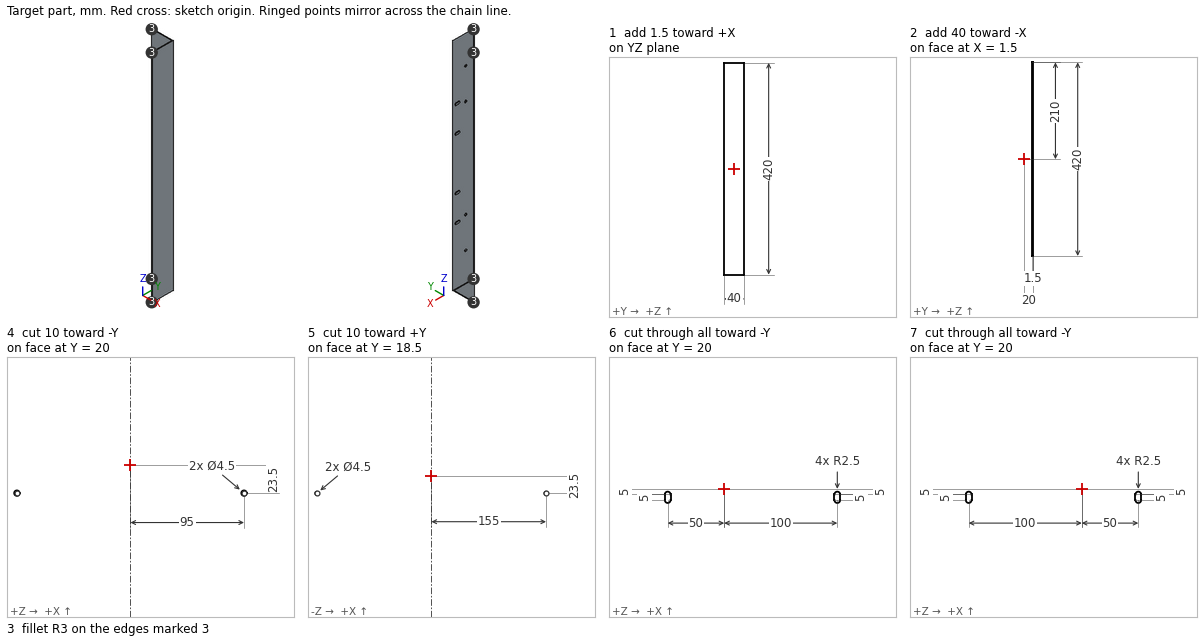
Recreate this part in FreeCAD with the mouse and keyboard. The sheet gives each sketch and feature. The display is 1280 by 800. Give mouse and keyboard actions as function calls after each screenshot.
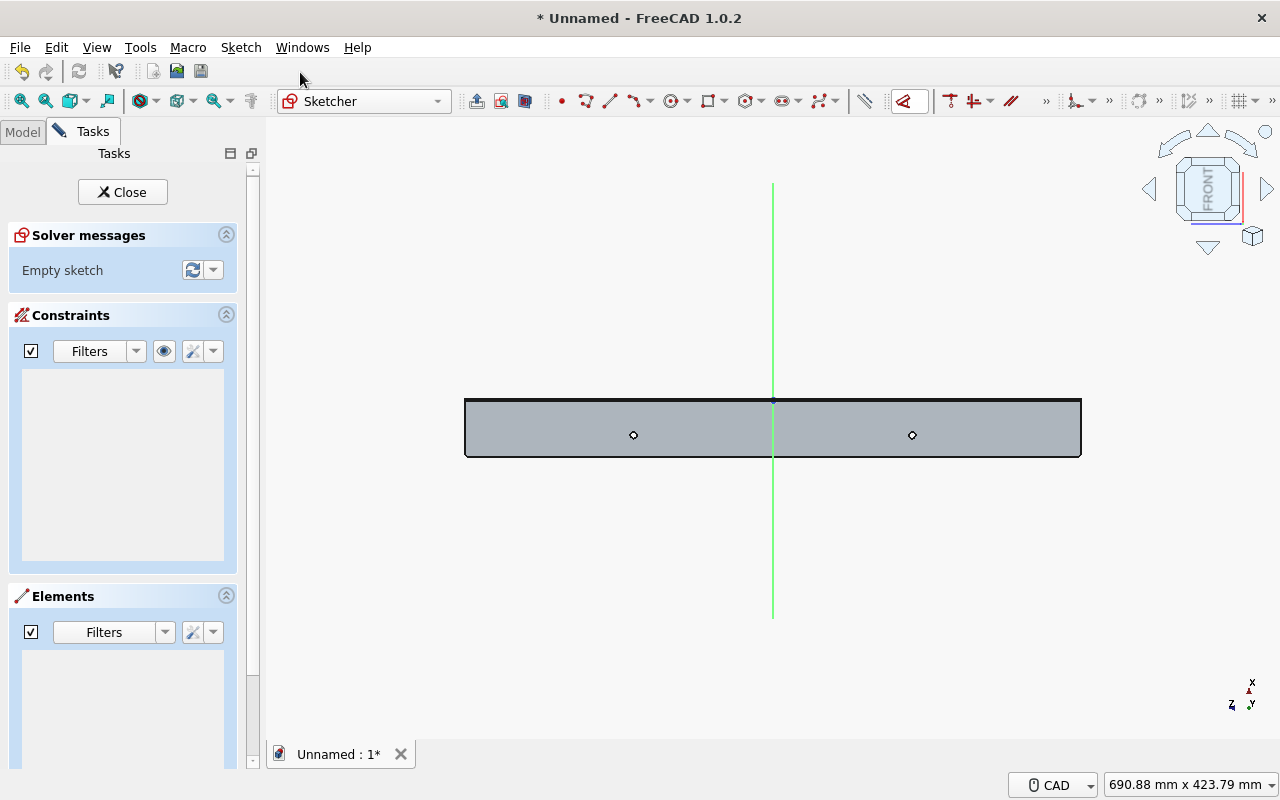
click(526, 102)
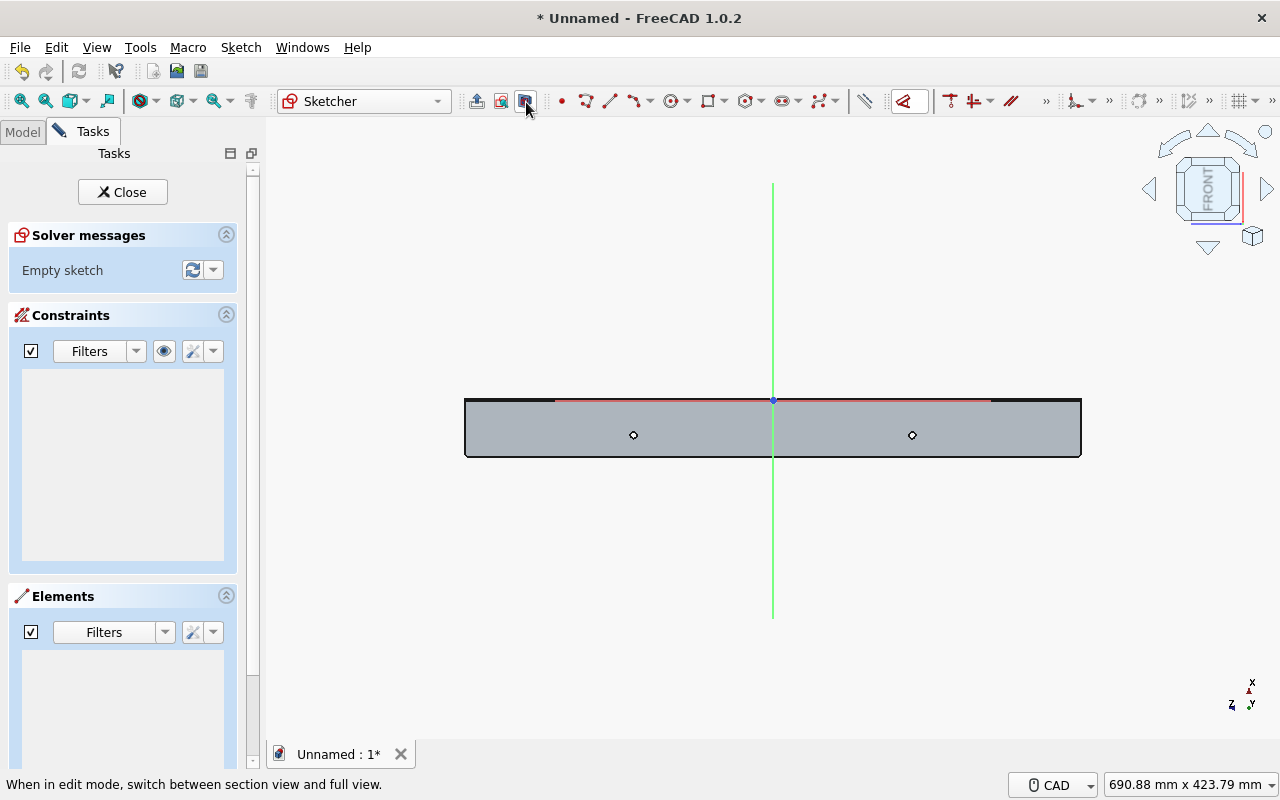
click(672, 102)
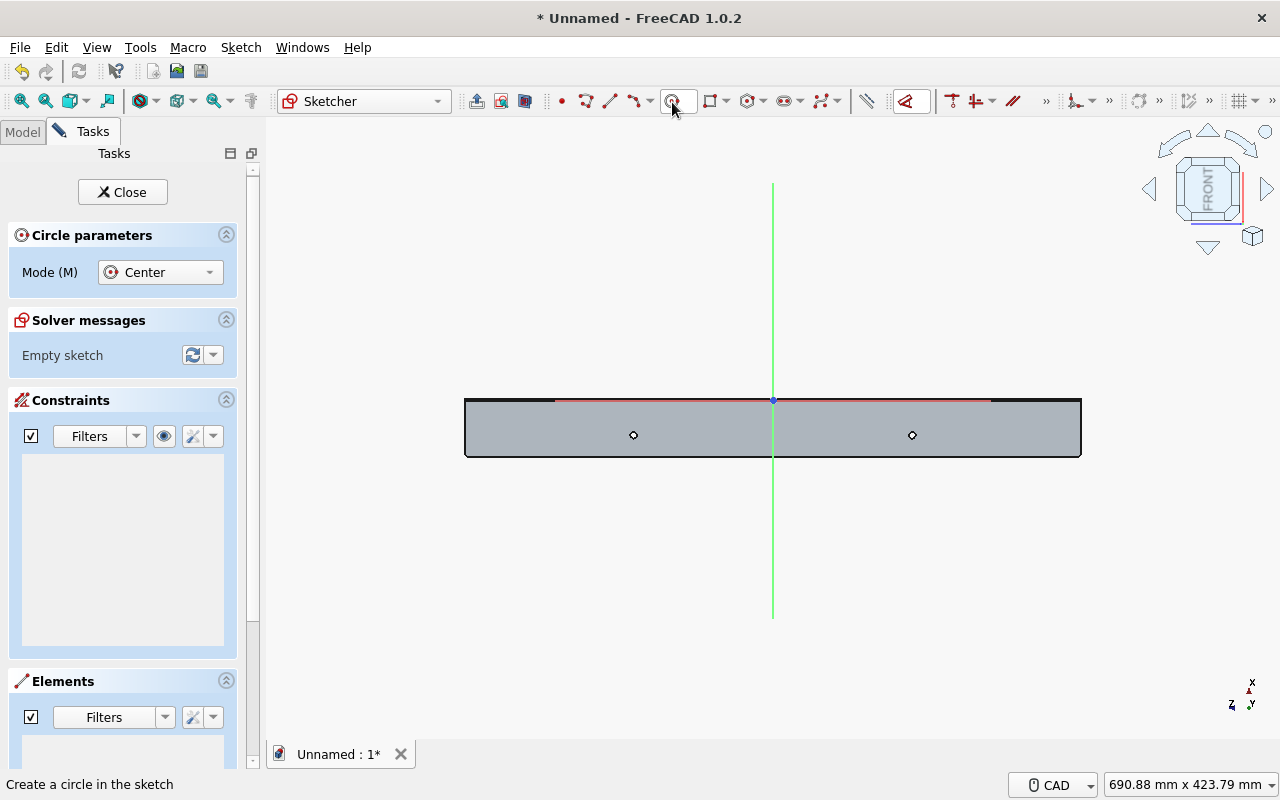
scroll(1000, 435, up, 10)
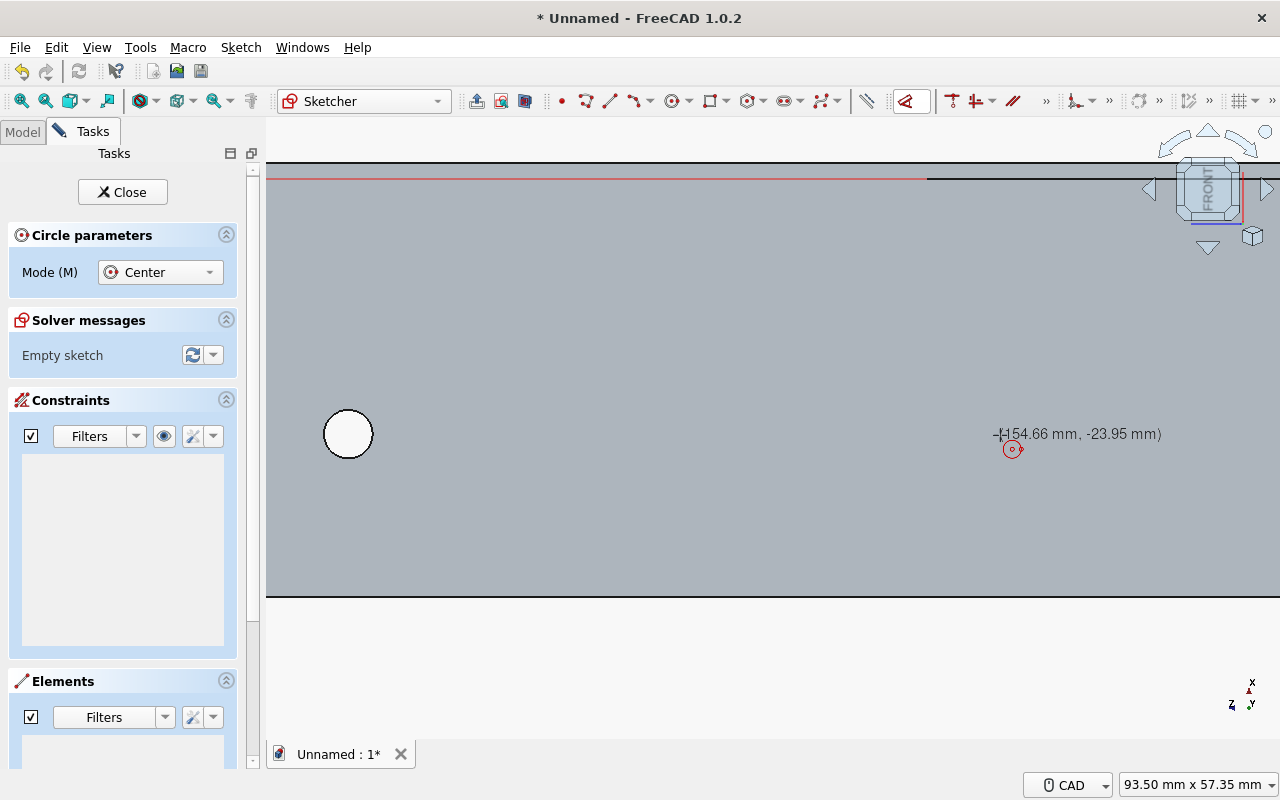
scroll(979, 450, down, 9)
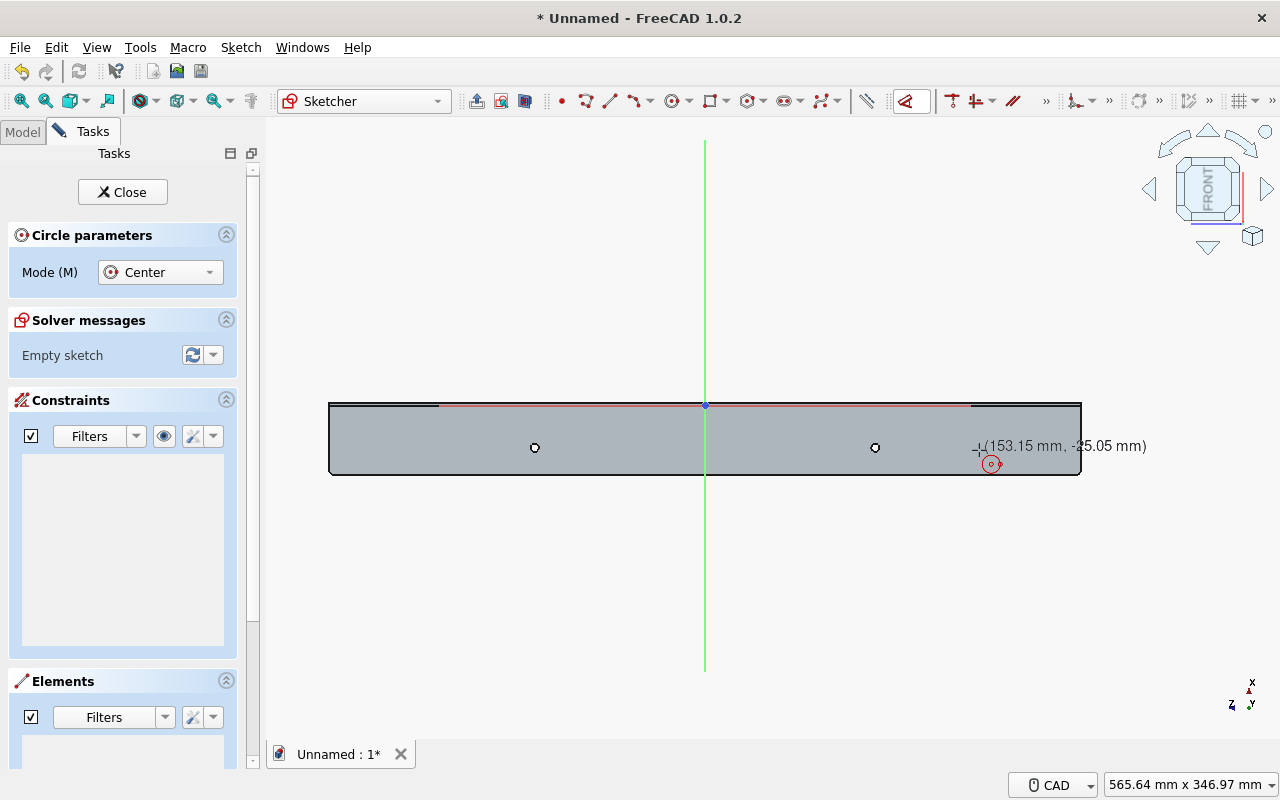
click(983, 448)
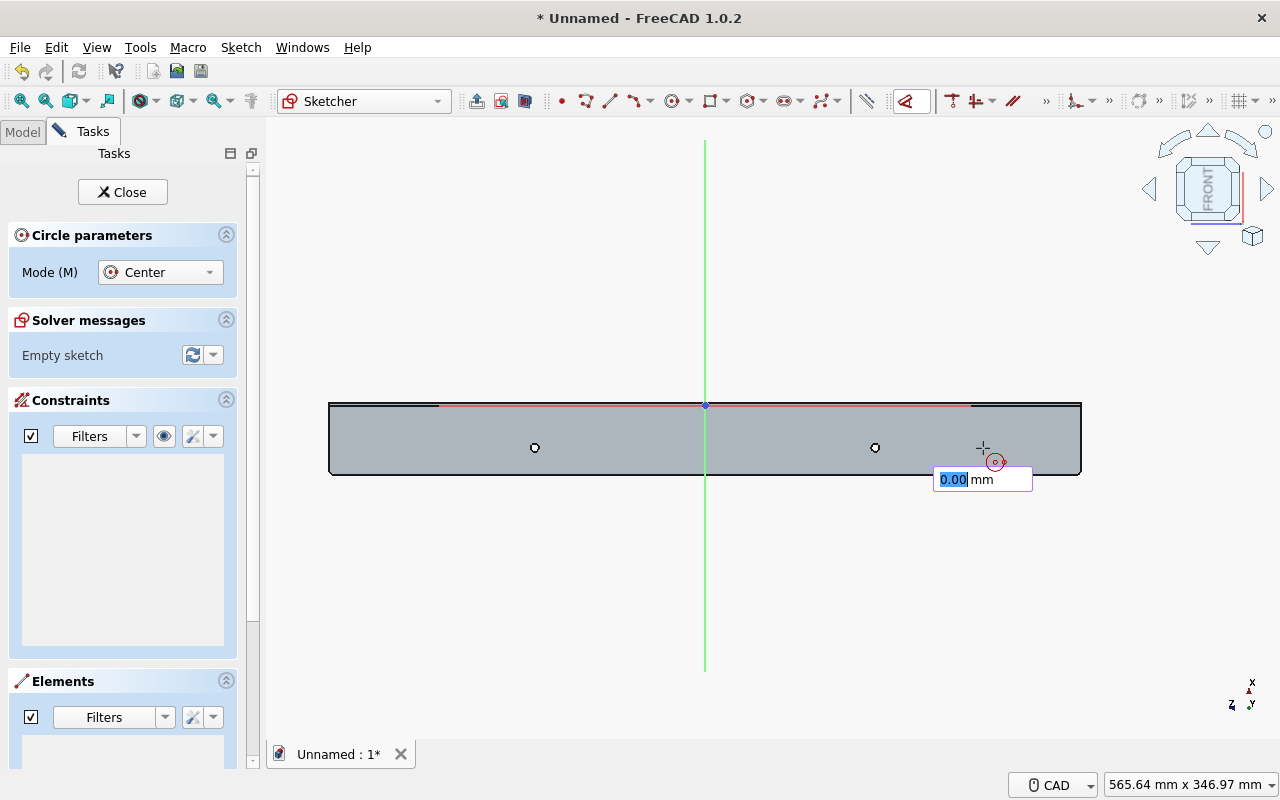
scroll(986, 445, up, 7)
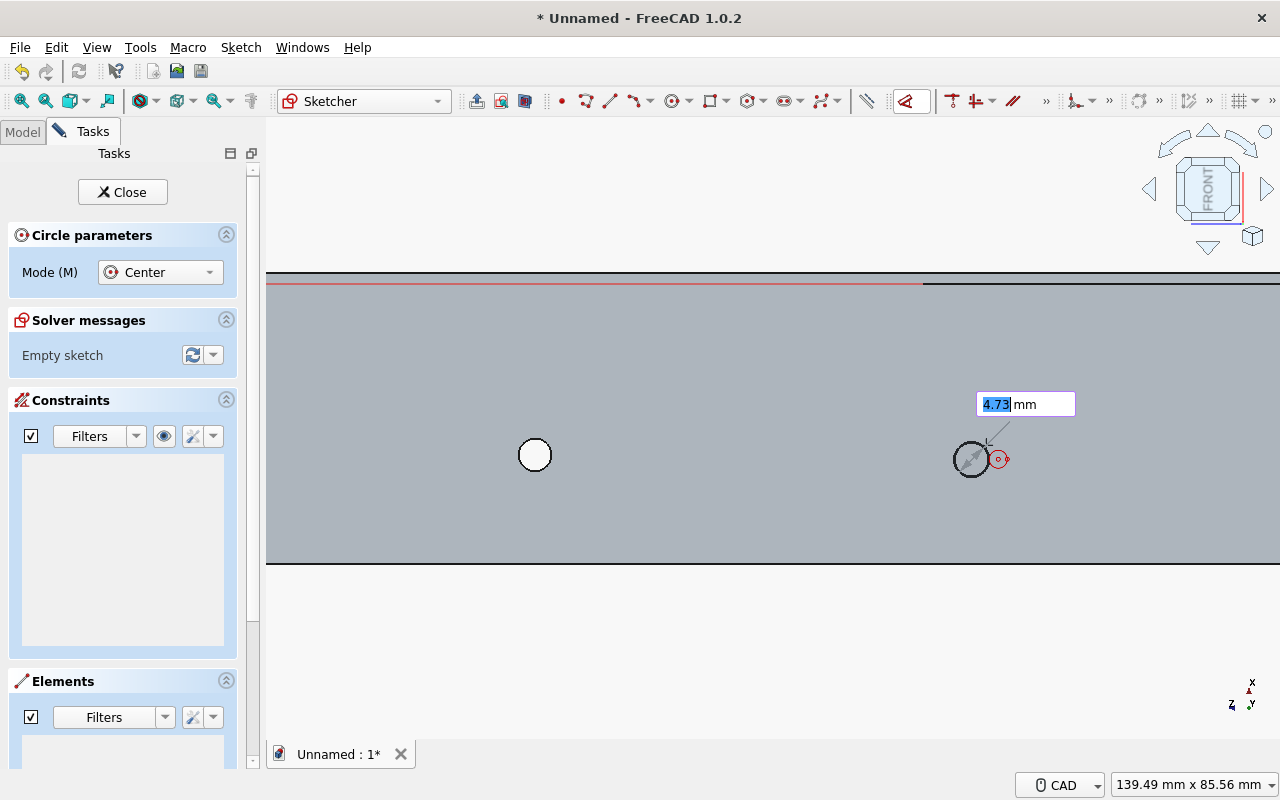
click(983, 443)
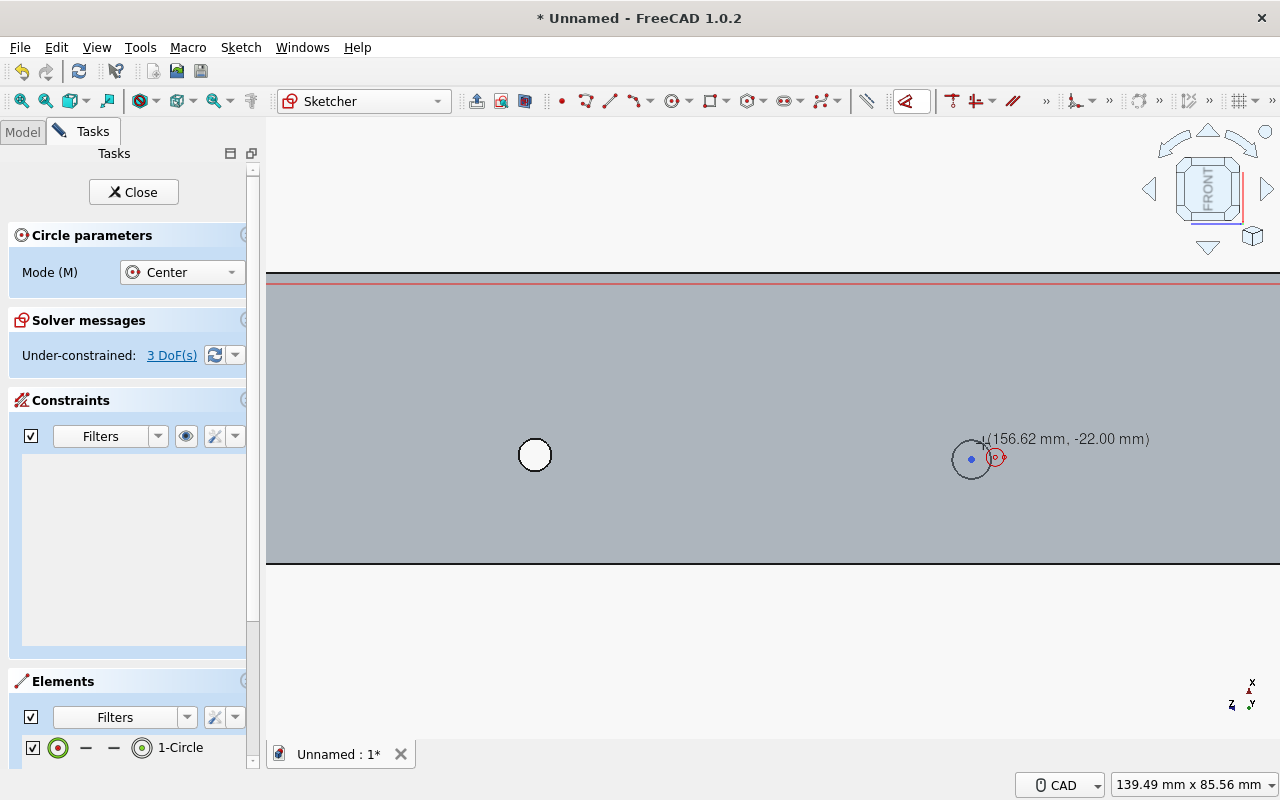
scroll(986, 444, down, 7)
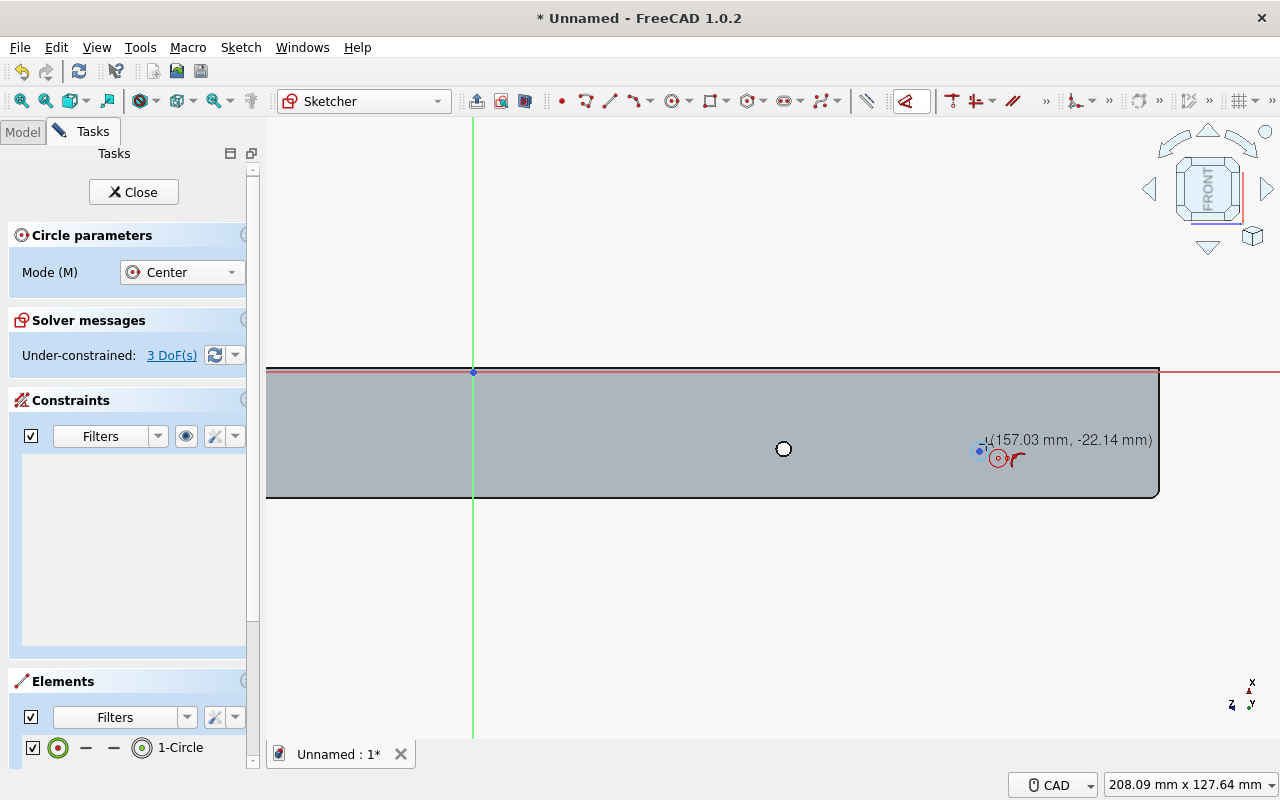
scroll(427, 447, up, 9)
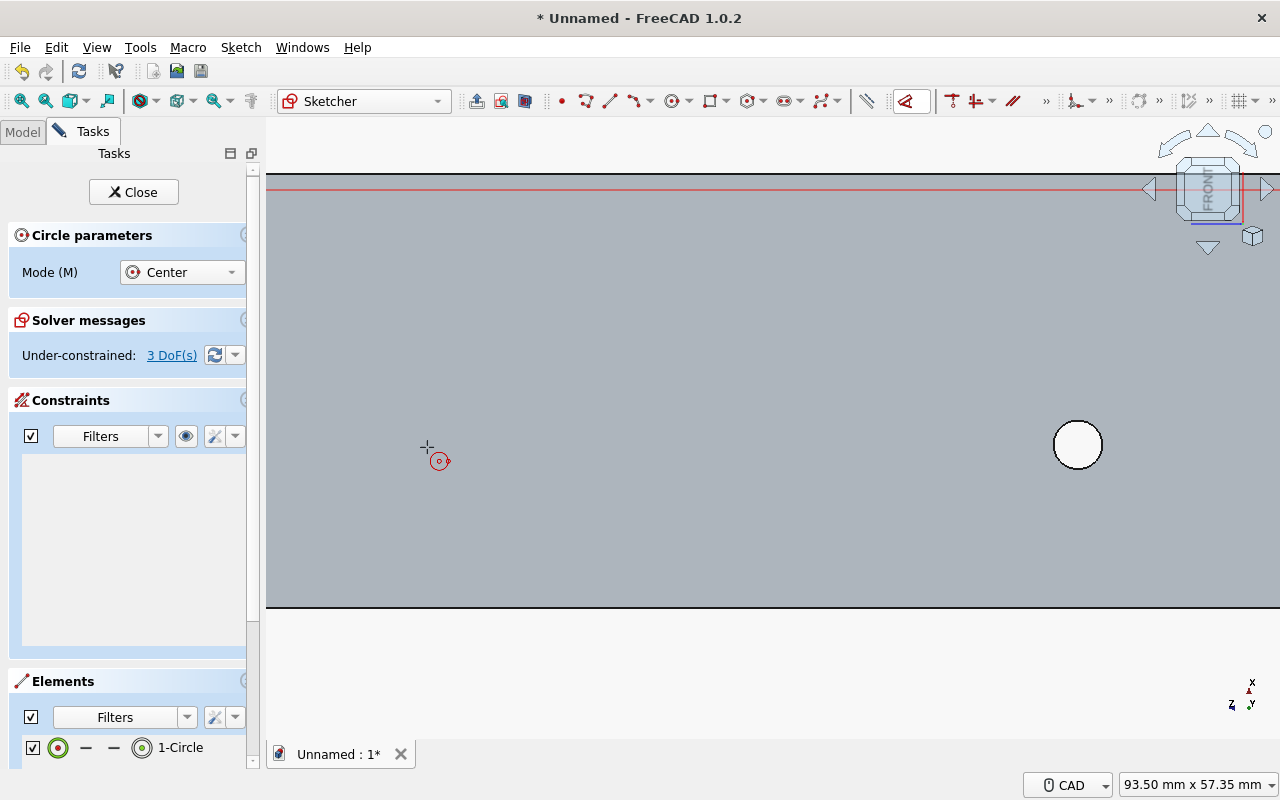
scroll(427, 447, down, 9)